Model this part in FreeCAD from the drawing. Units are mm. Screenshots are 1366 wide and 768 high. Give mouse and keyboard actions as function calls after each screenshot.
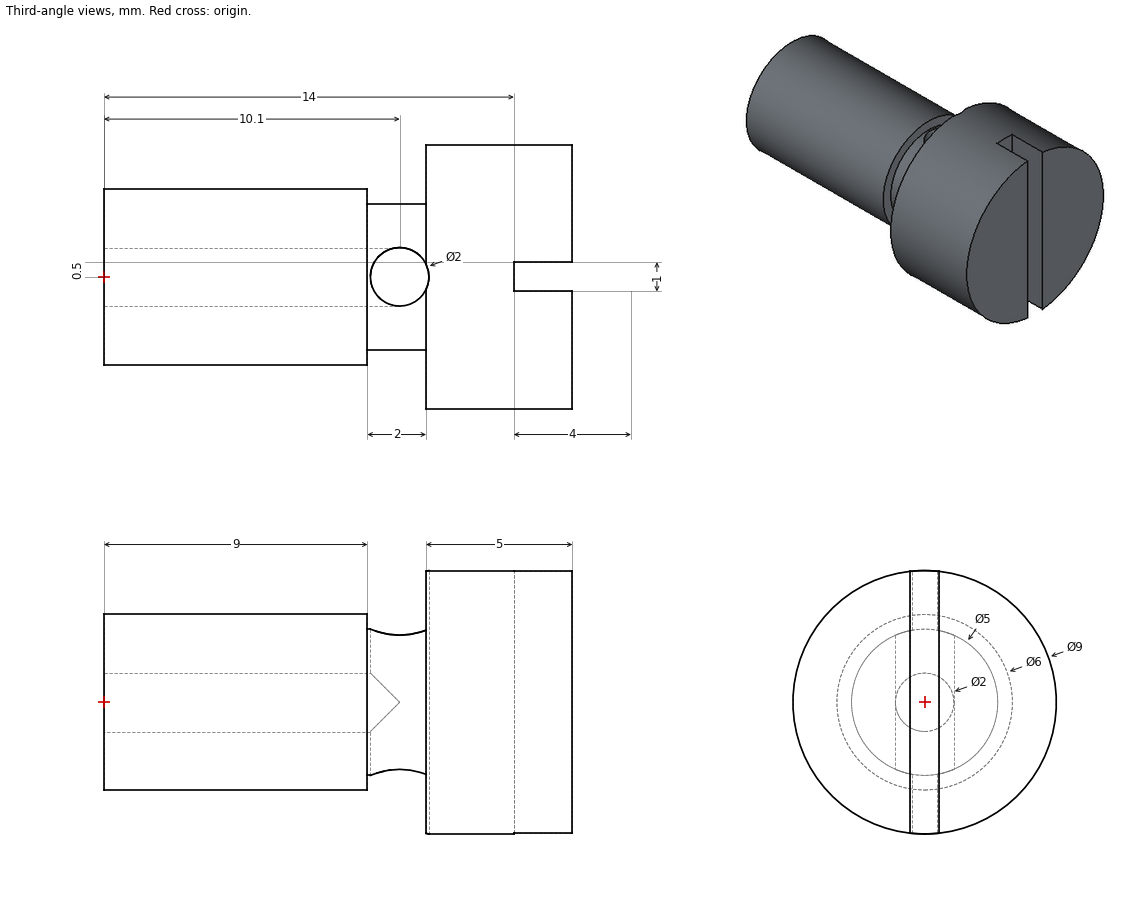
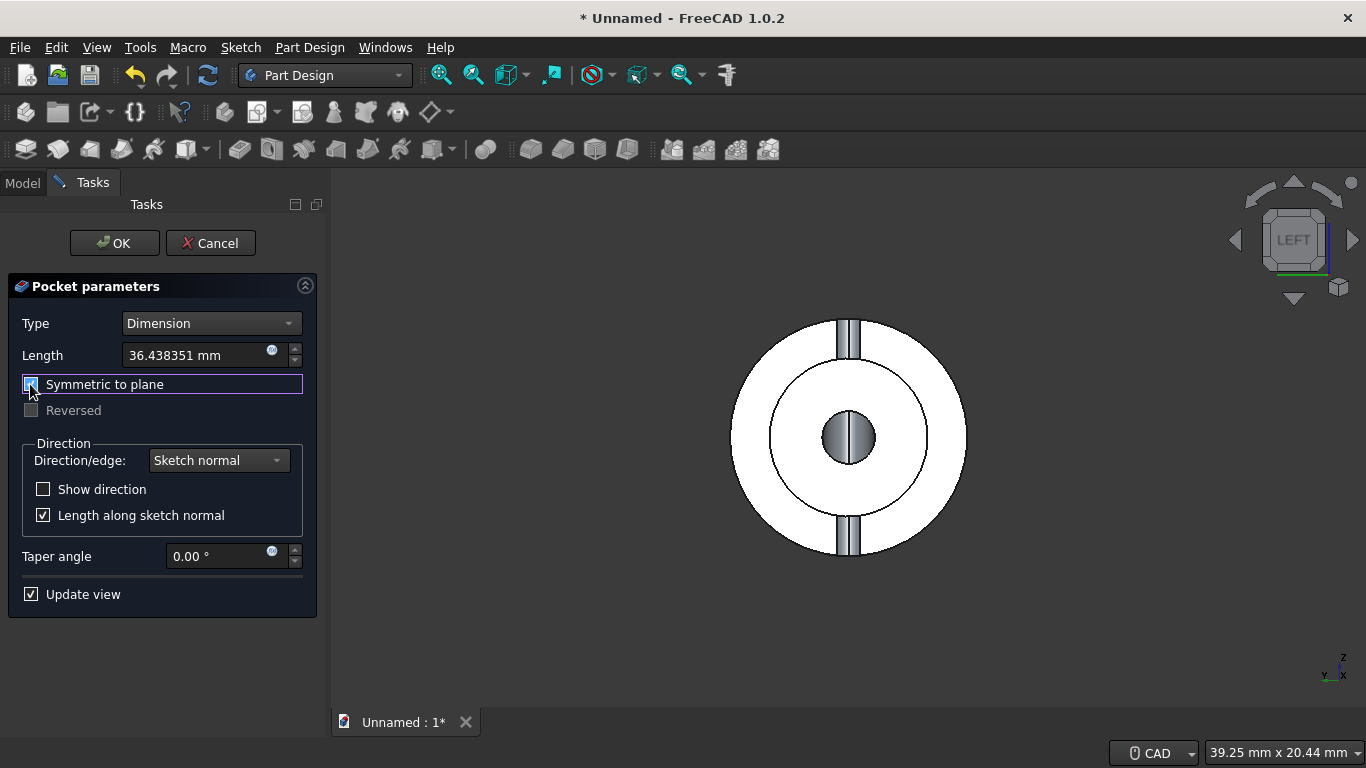
click(115, 243)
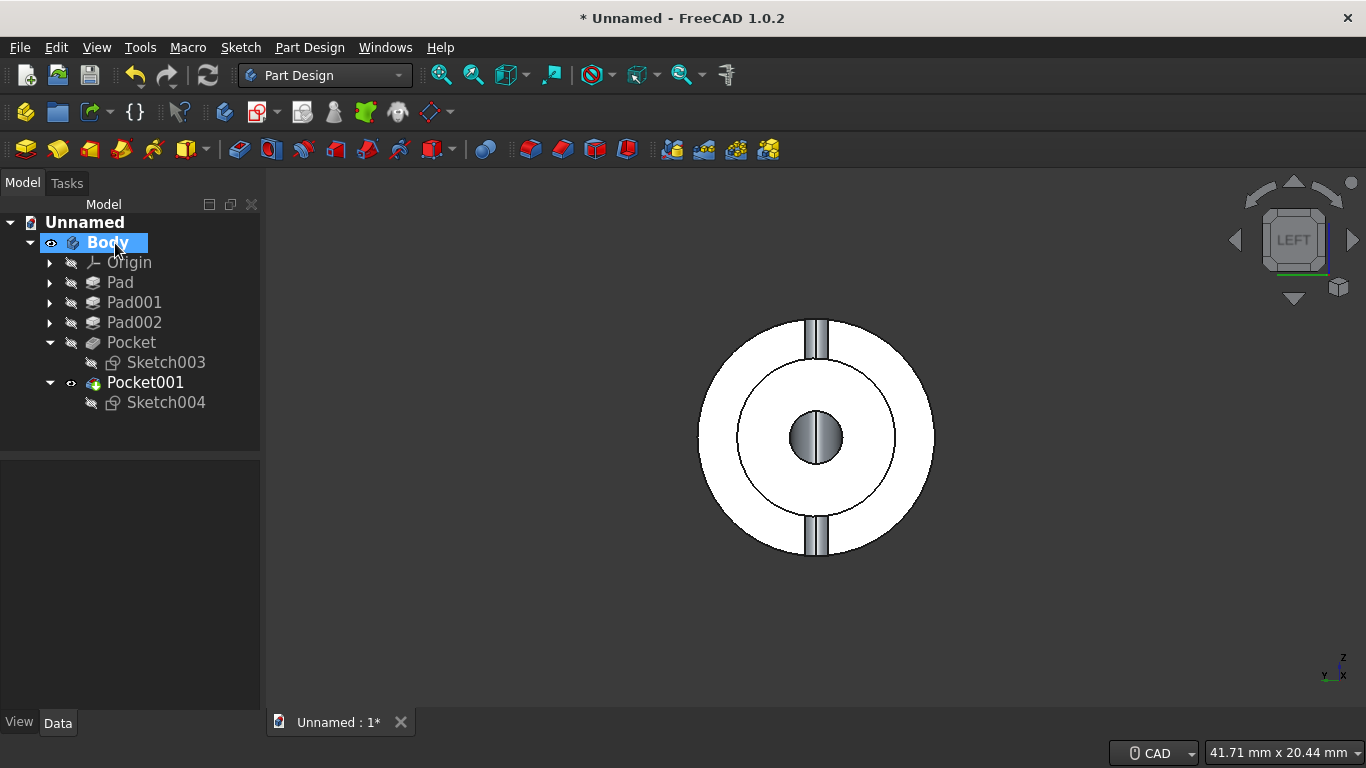
key(v)
key(f)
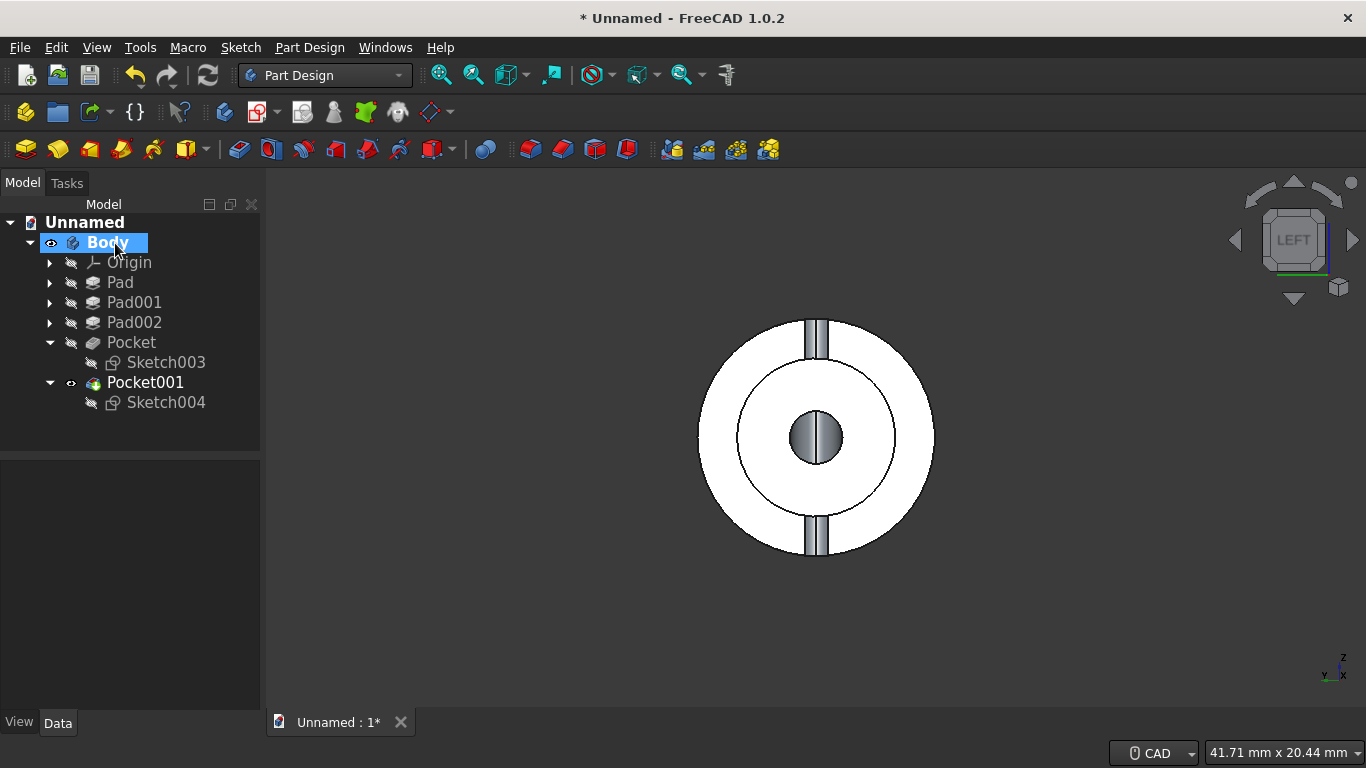
click(258, 112)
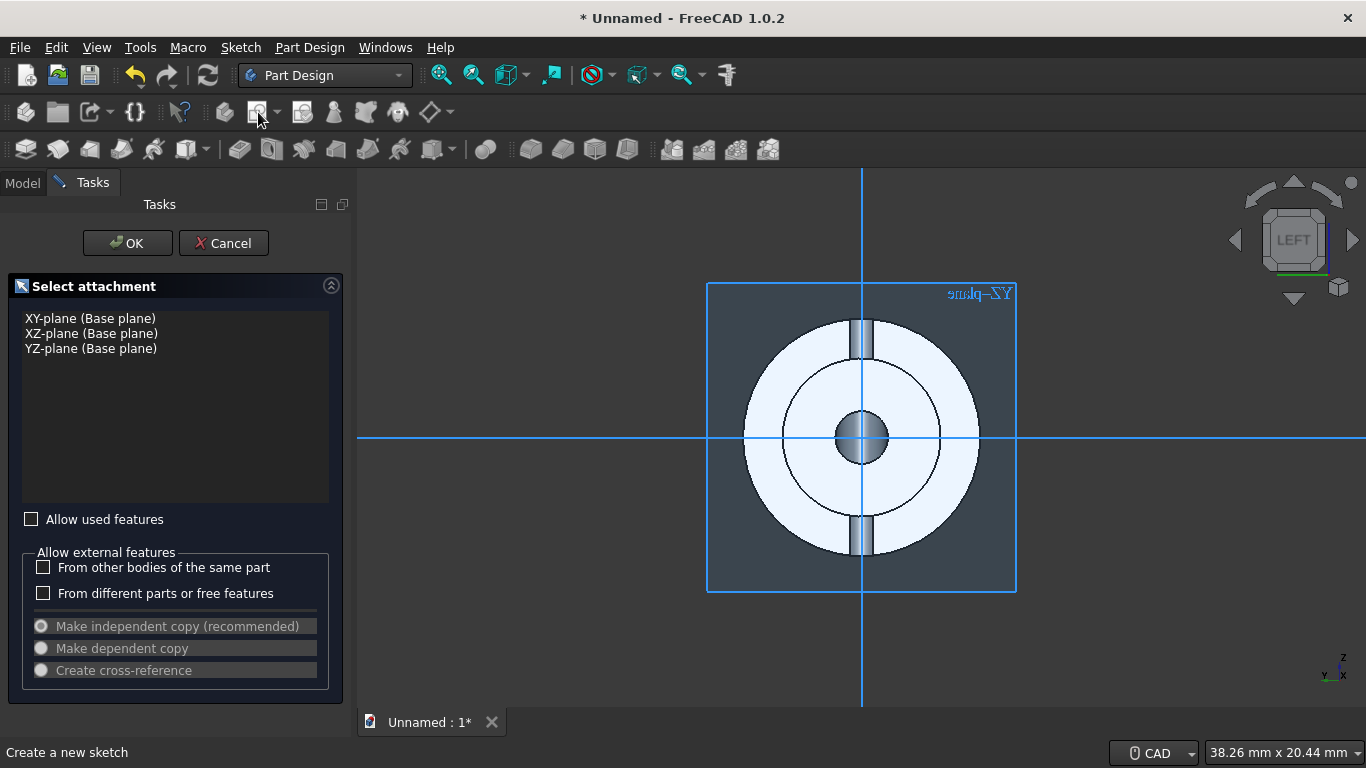
click(82, 318)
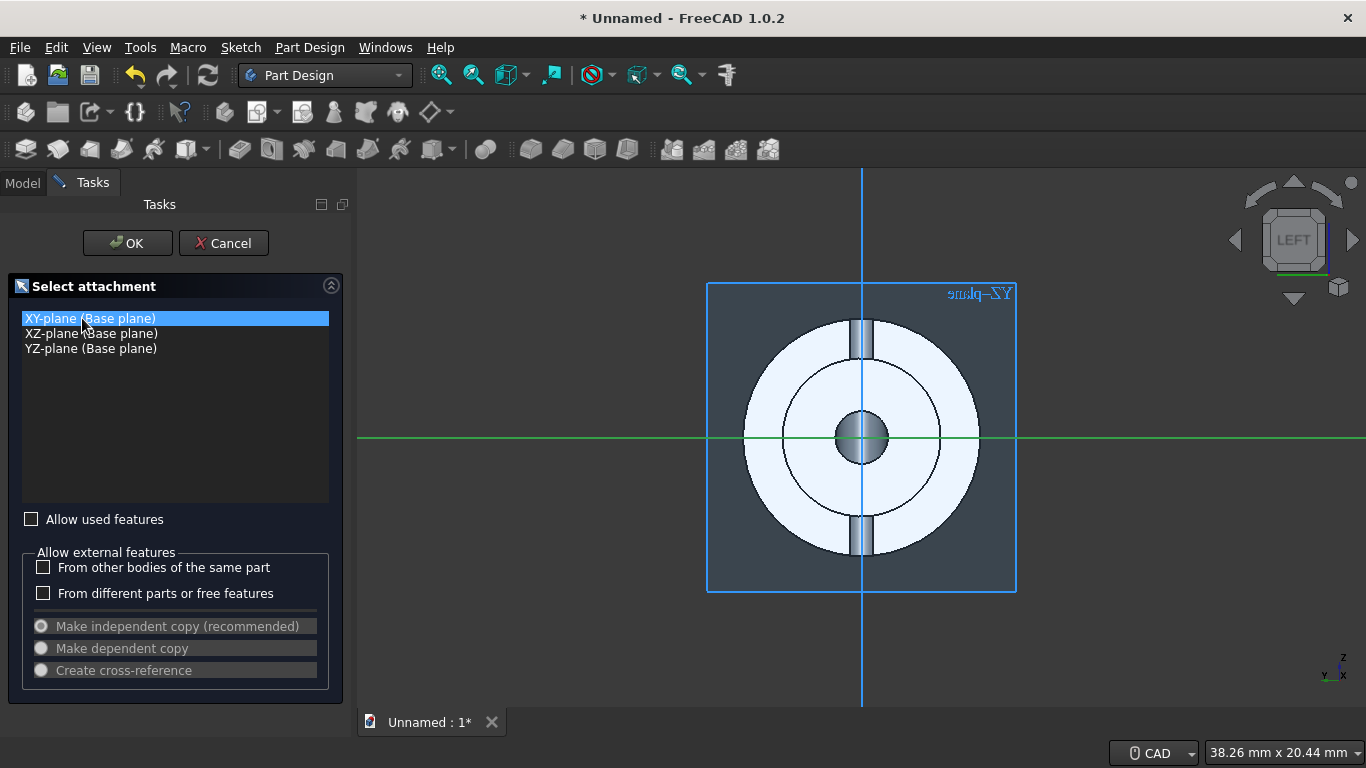
click(128, 243)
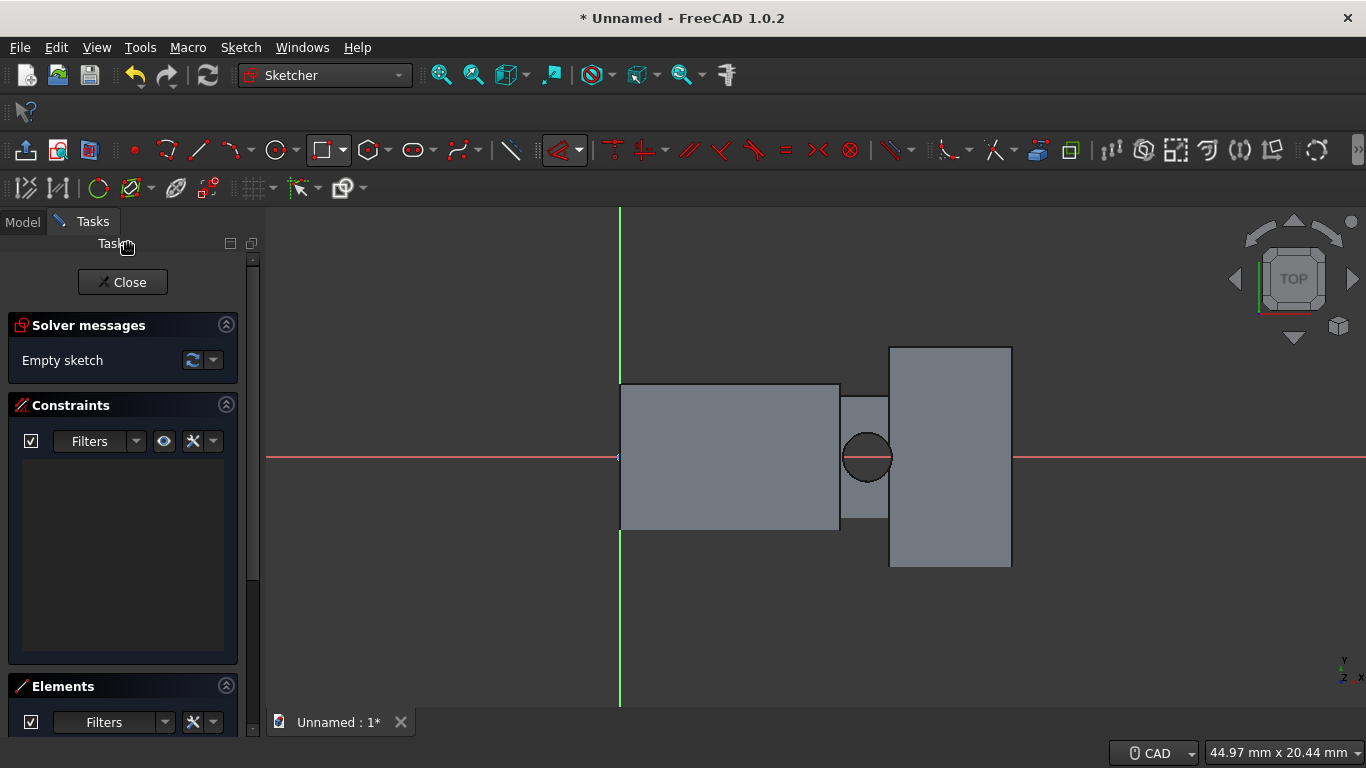
click(90, 150)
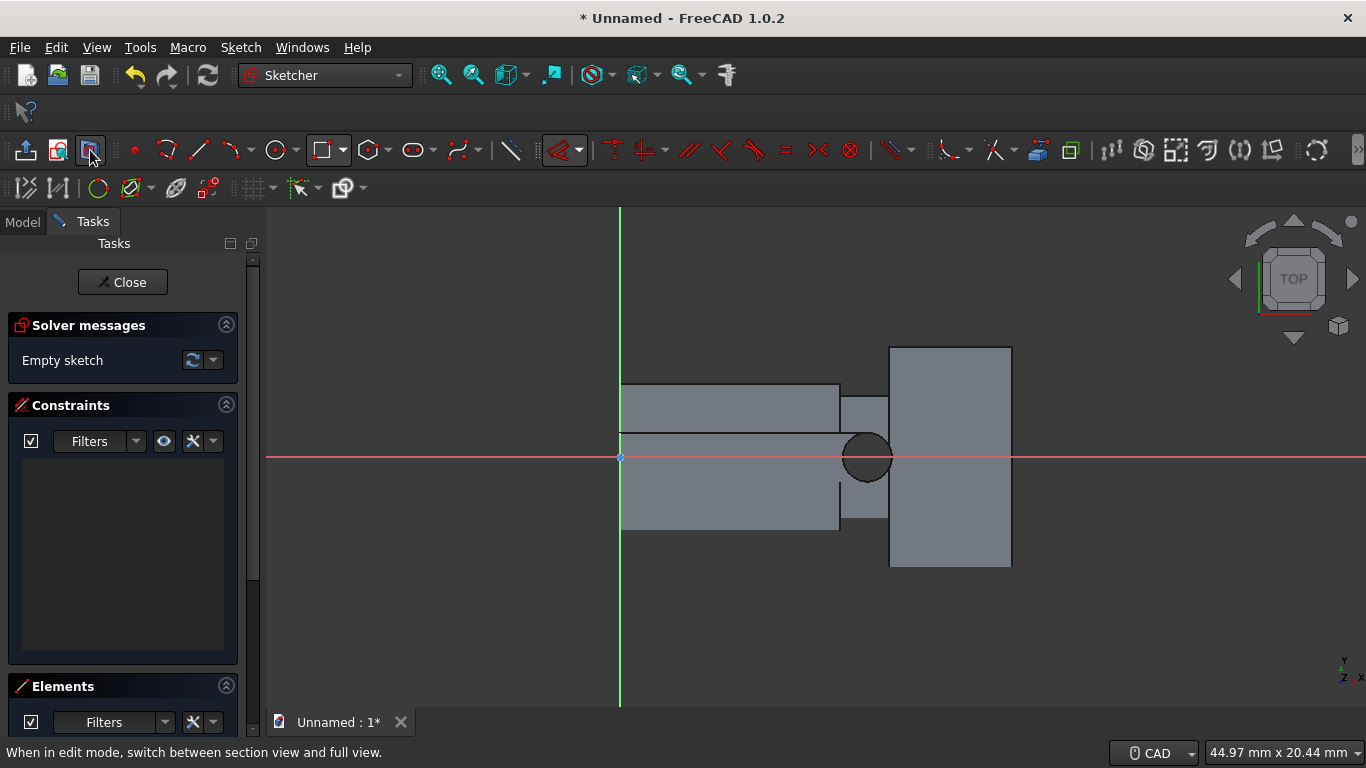
scroll(1064, 457, up, 9)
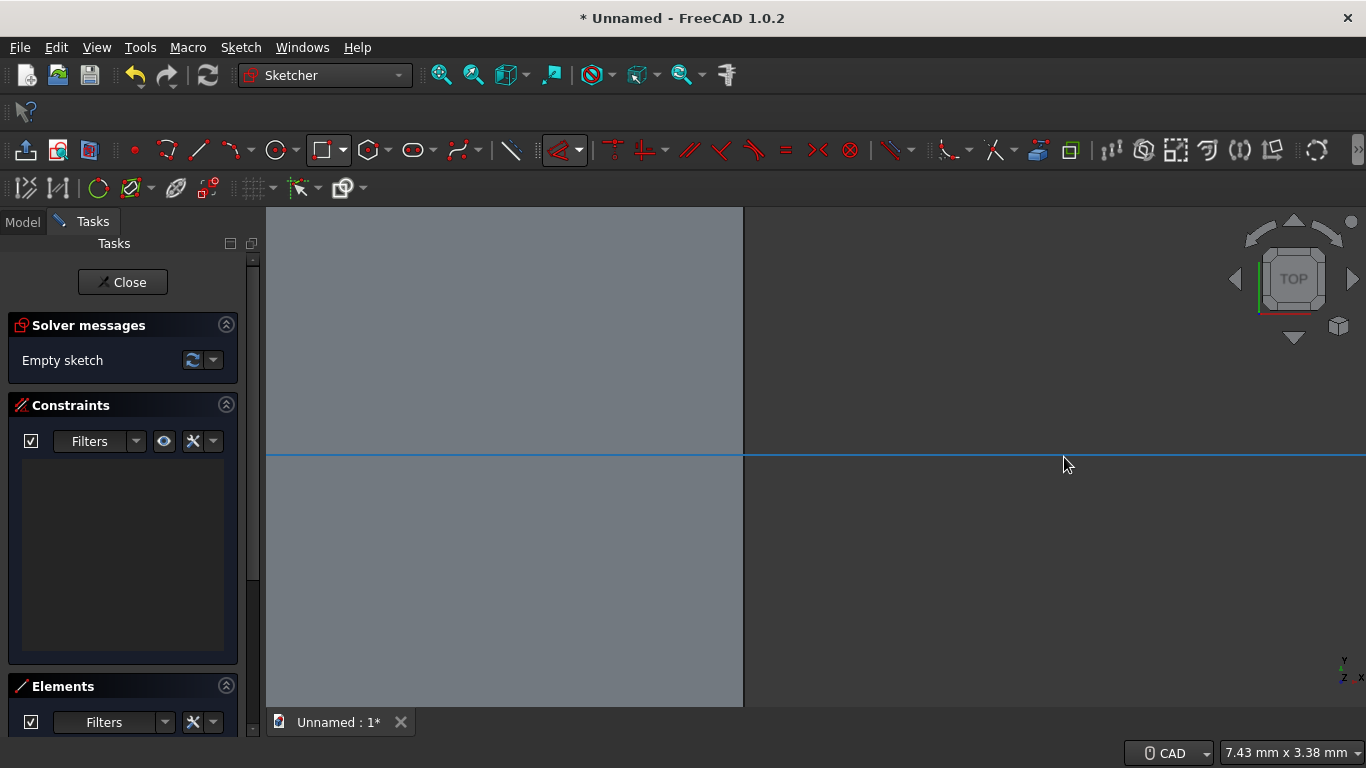
key(g)
key(r)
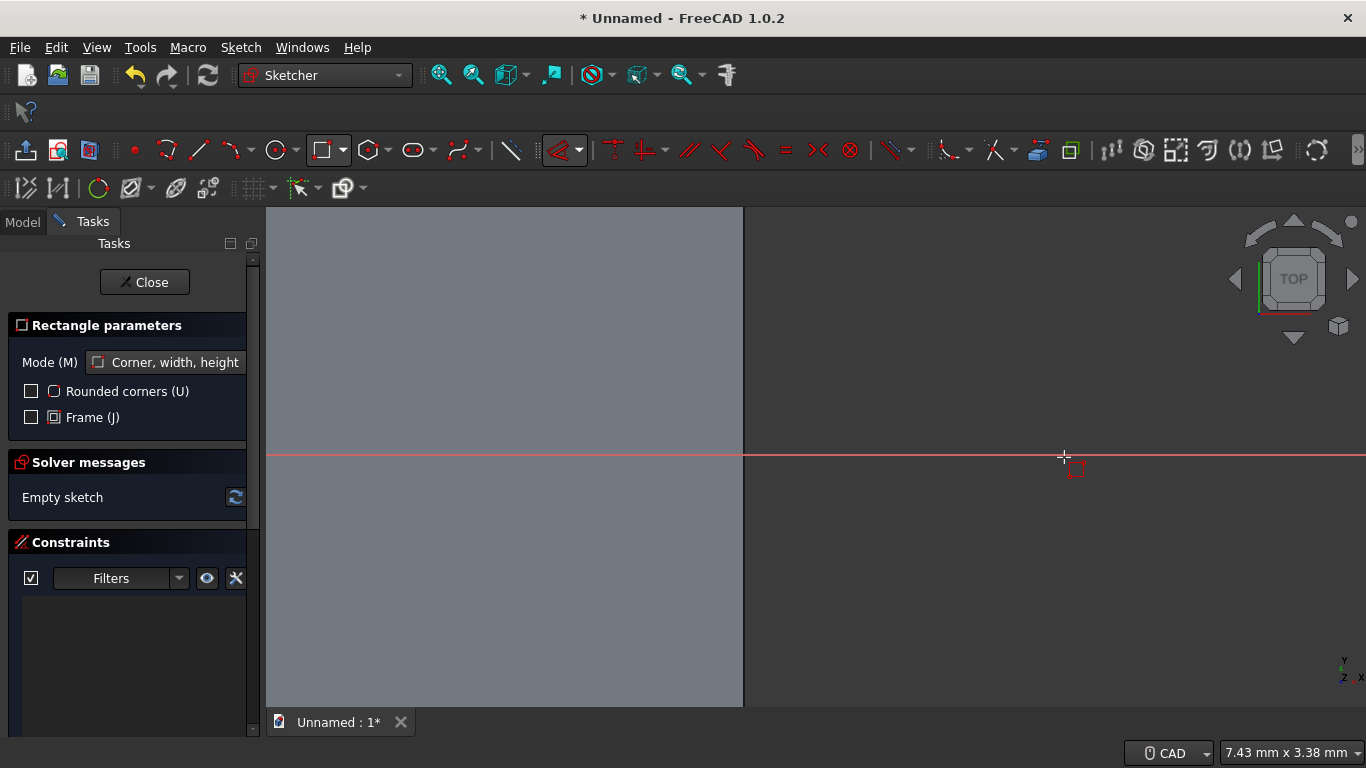
click(448, 381)
click(1040, 529)
key(Escape)